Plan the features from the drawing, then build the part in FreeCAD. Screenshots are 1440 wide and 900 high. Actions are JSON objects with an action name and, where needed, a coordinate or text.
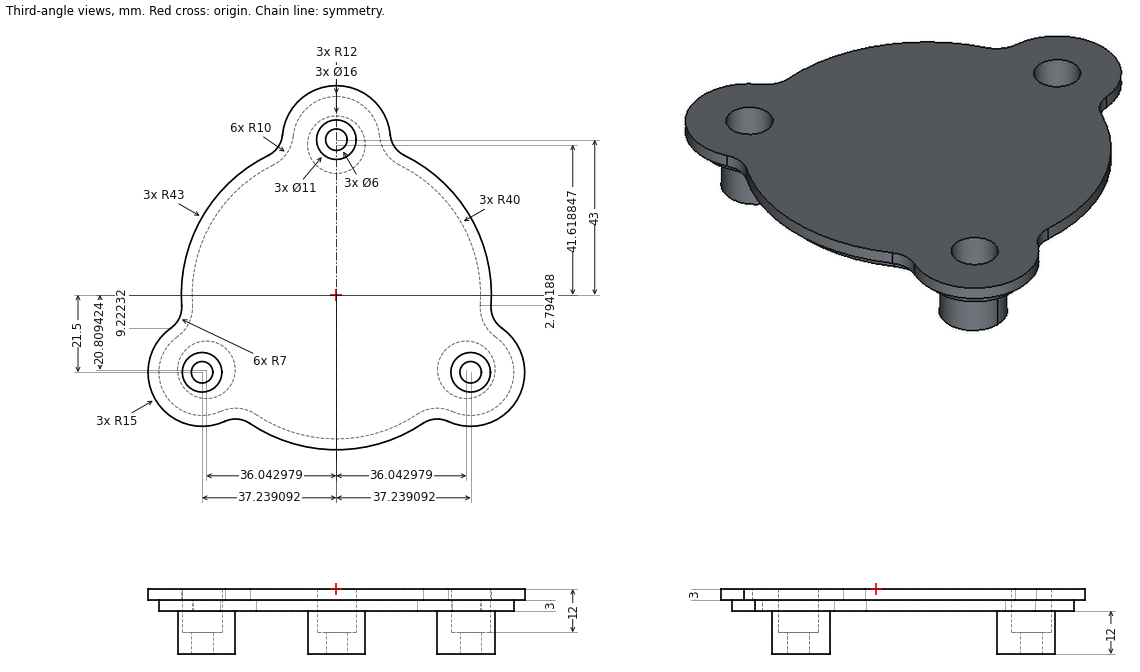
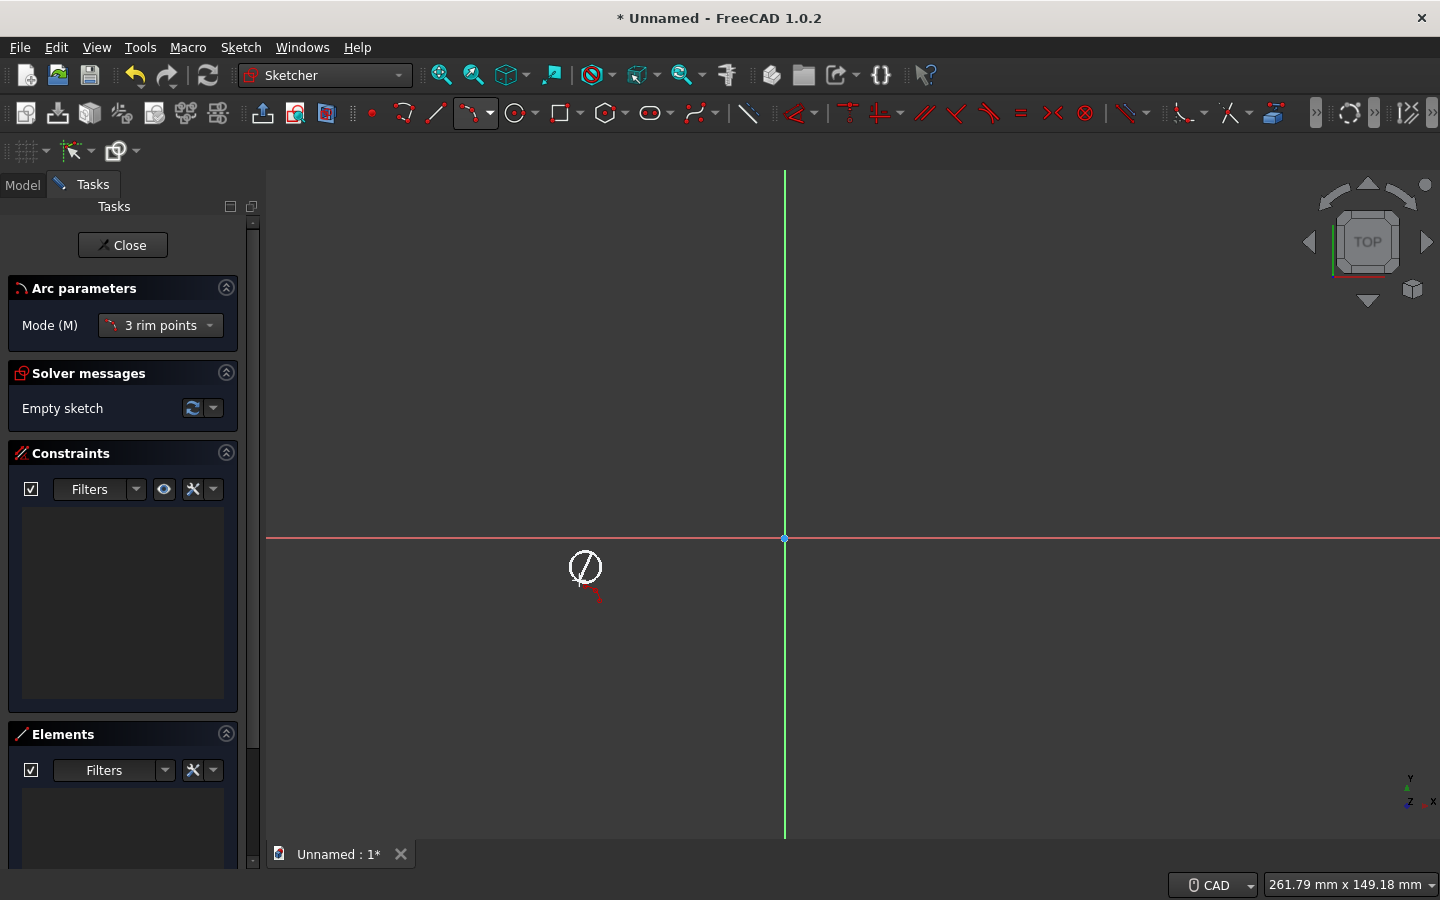
{"action": "scroll", "coordinate": [589, 568], "scroll_direction": "up", "scroll_amount": 7}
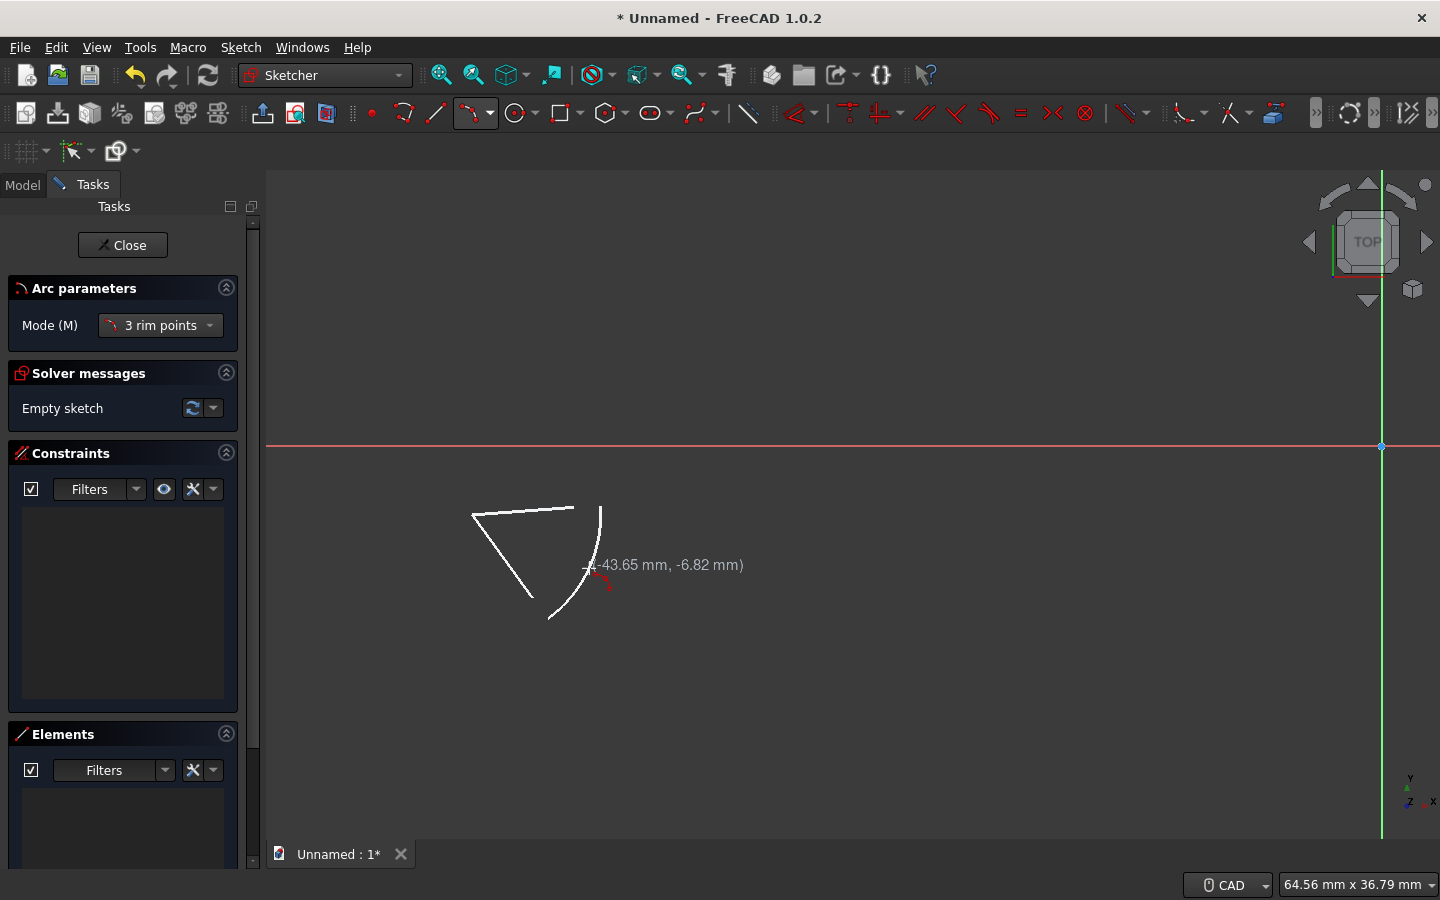
{"action": "left_click", "coordinate": [590, 564]}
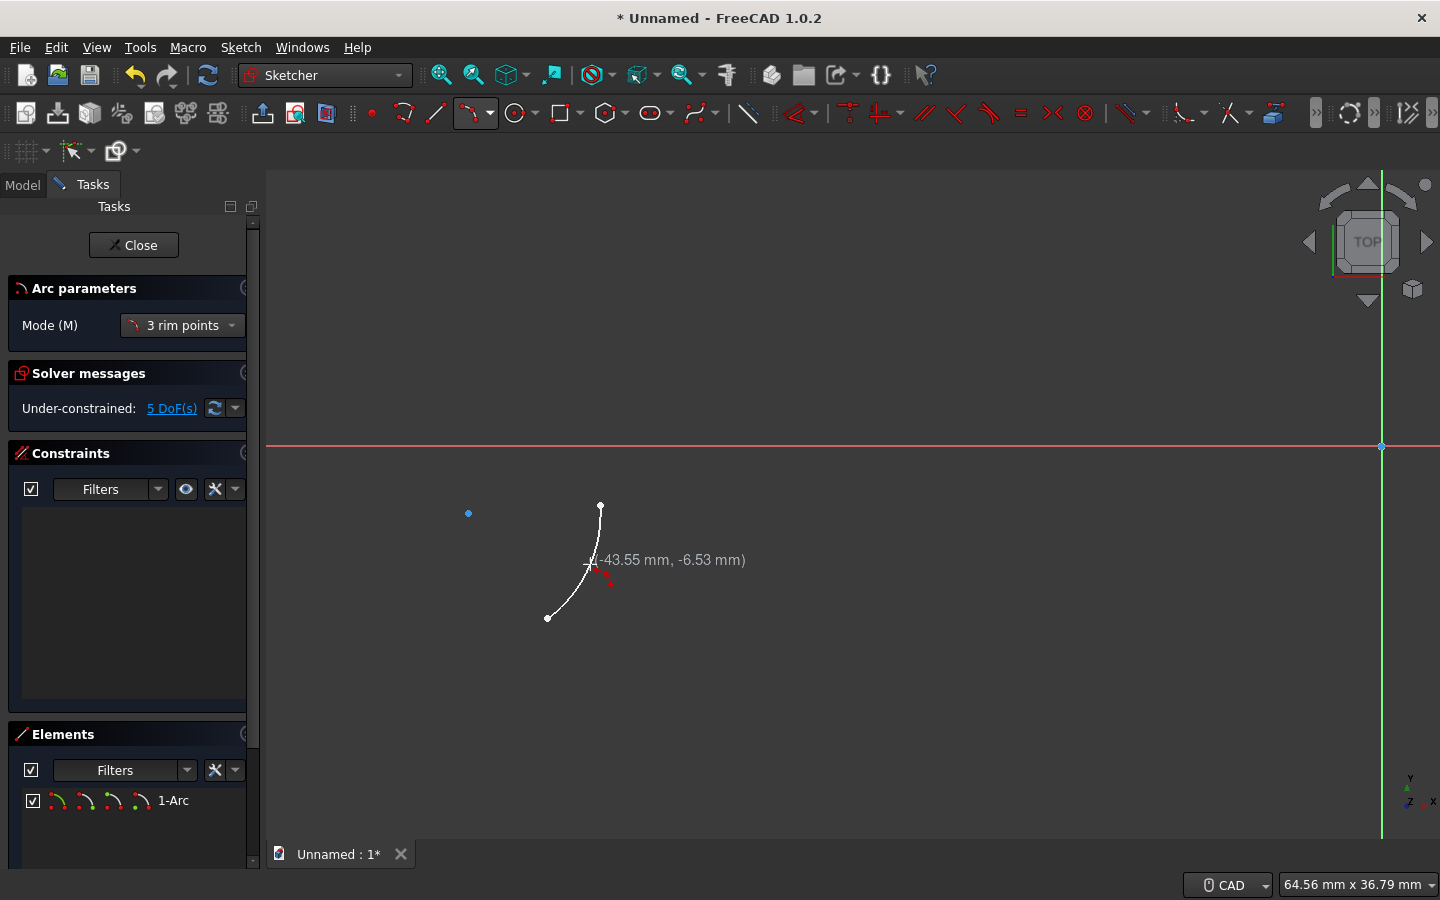
{"action": "scroll", "coordinate": [589, 568], "scroll_direction": "down", "scroll_amount": 7}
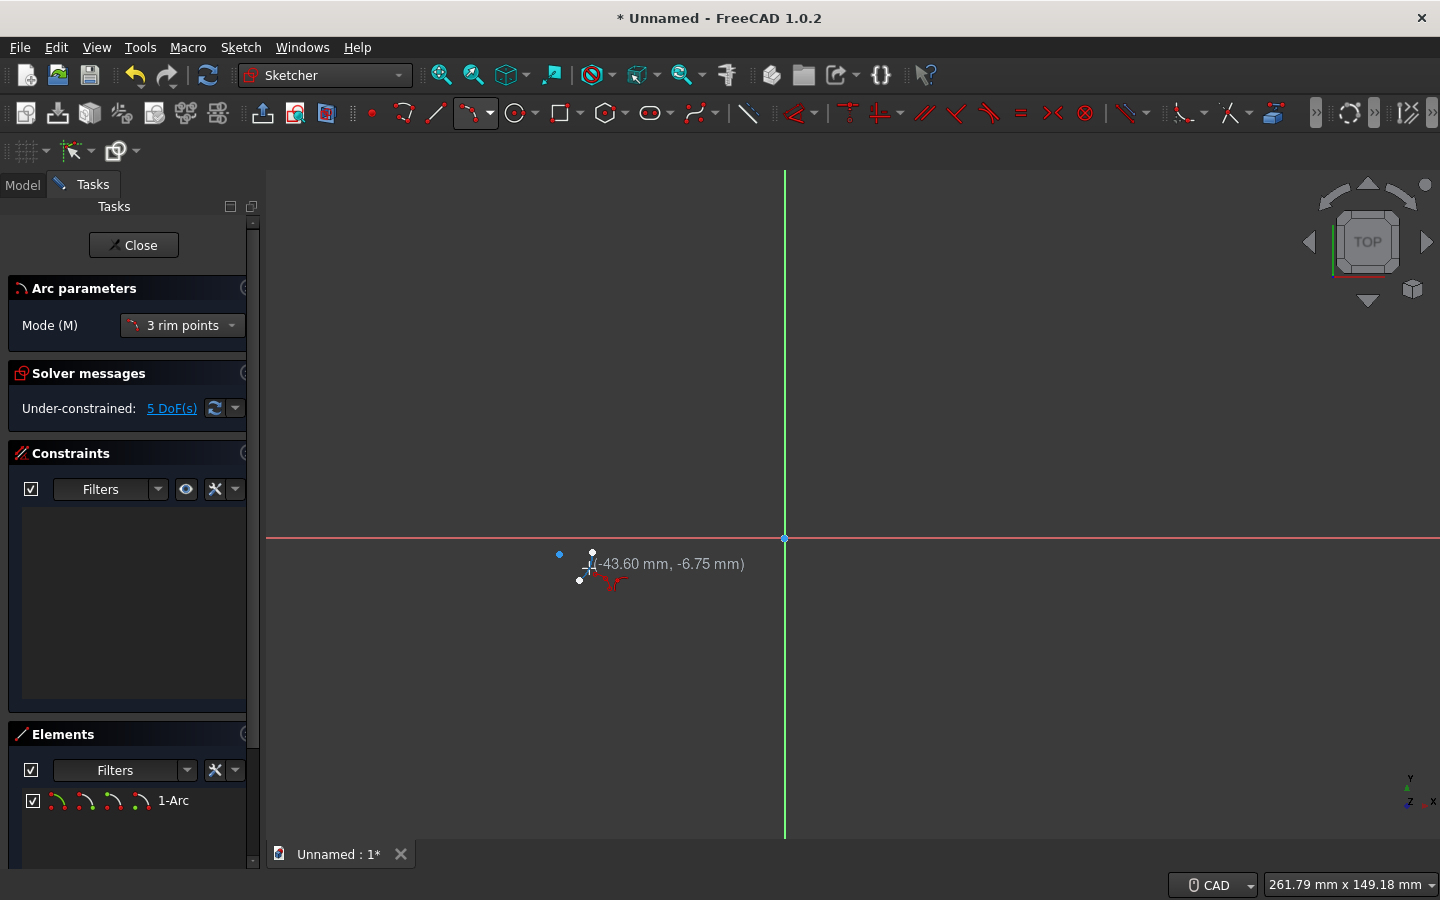
{"action": "left_click", "coordinate": [579, 581]}
{"action": "left_click", "coordinate": [646, 696]}
{"action": "left_click", "coordinate": [559, 668]}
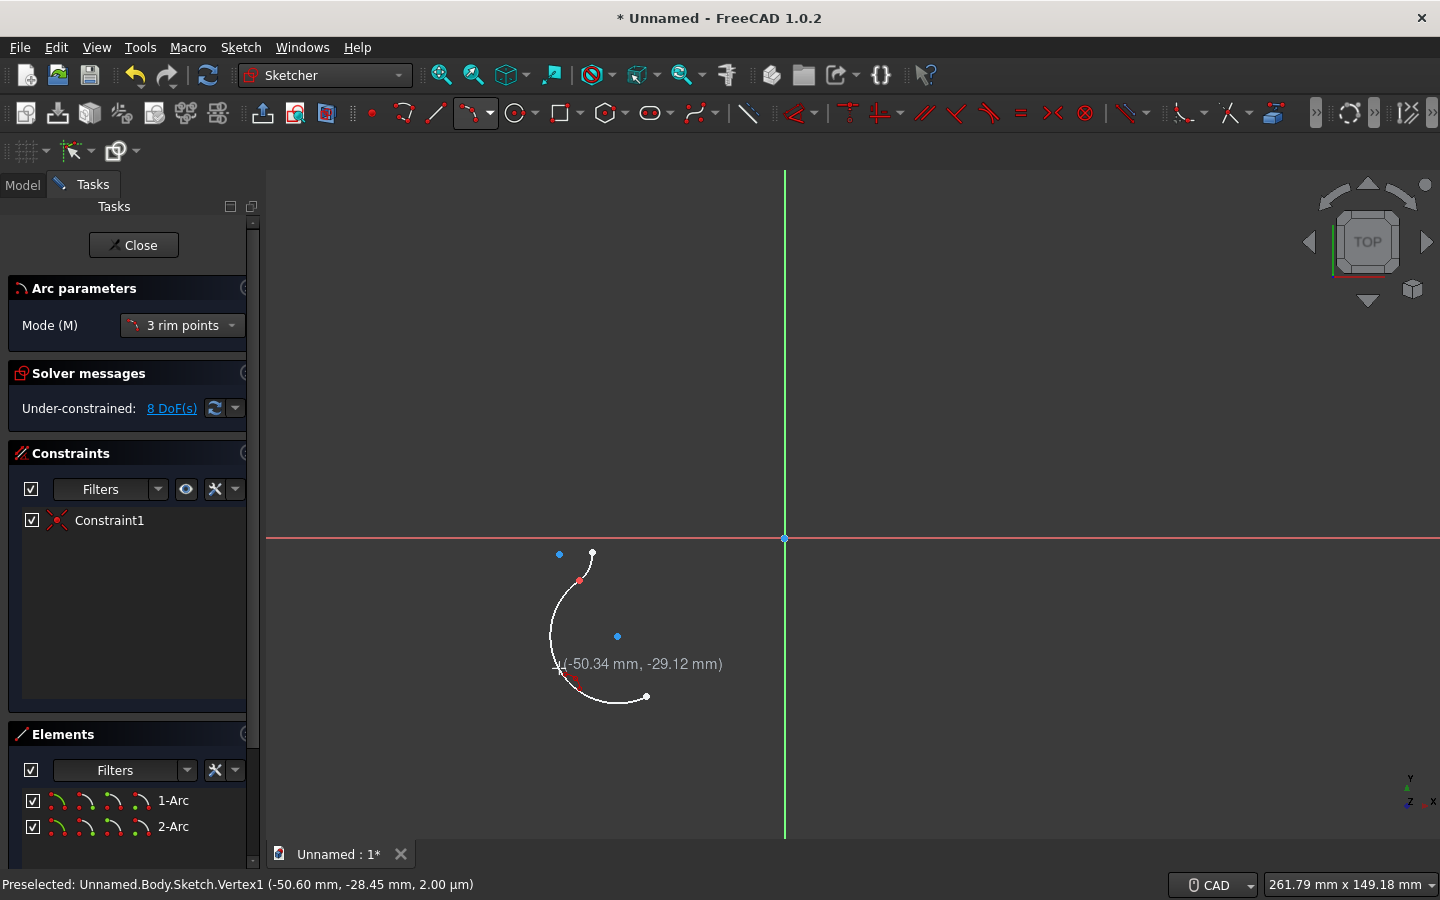
{"action": "left_click", "coordinate": [646, 697]}
{"action": "left_click", "coordinate": [677, 698]}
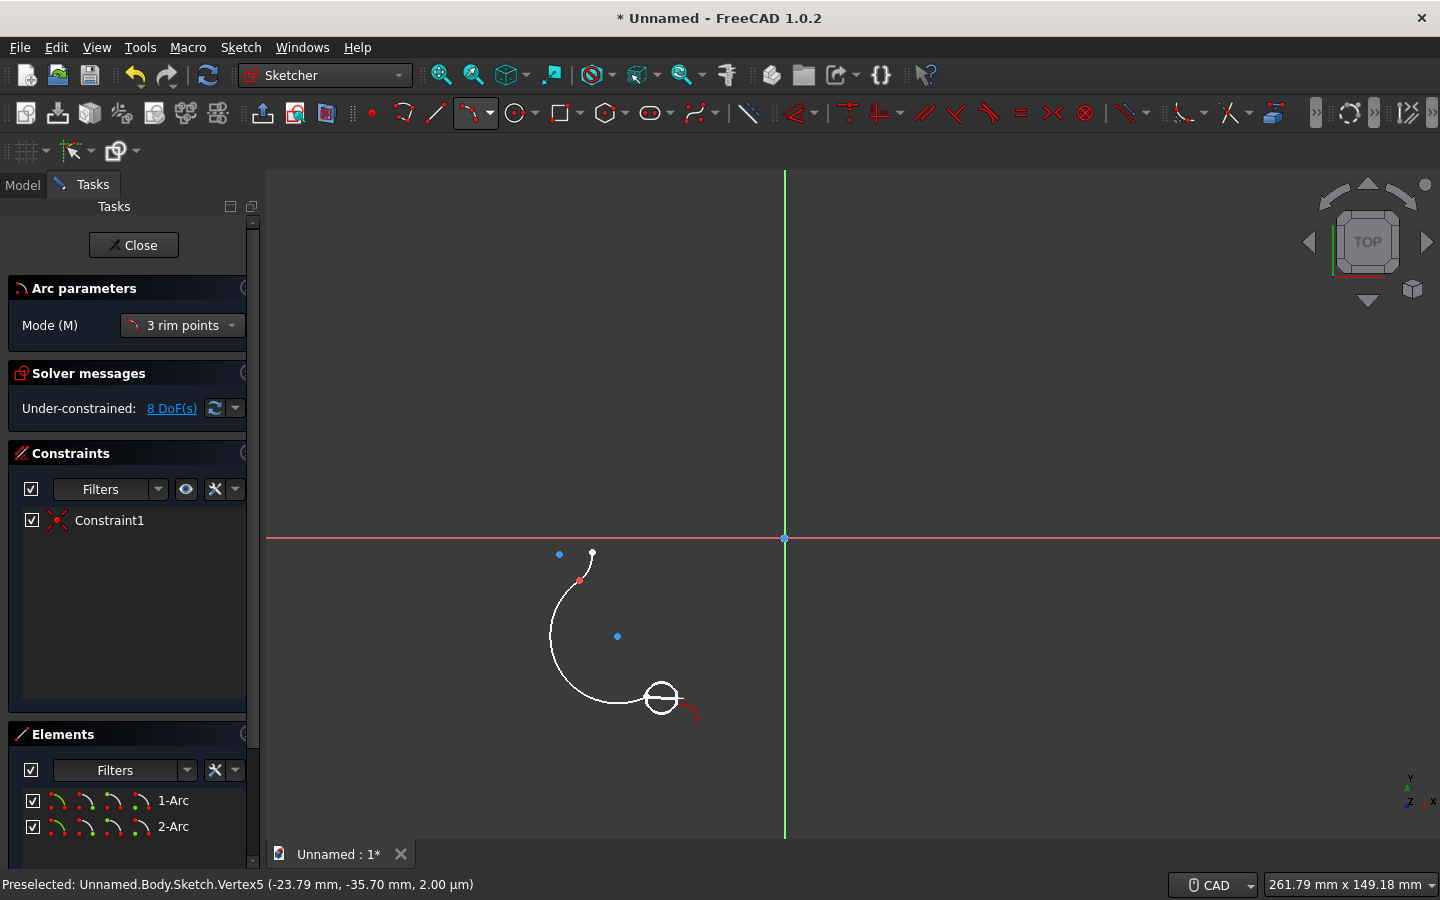
{"action": "scroll", "coordinate": [662, 693], "scroll_direction": "up", "scroll_amount": 7}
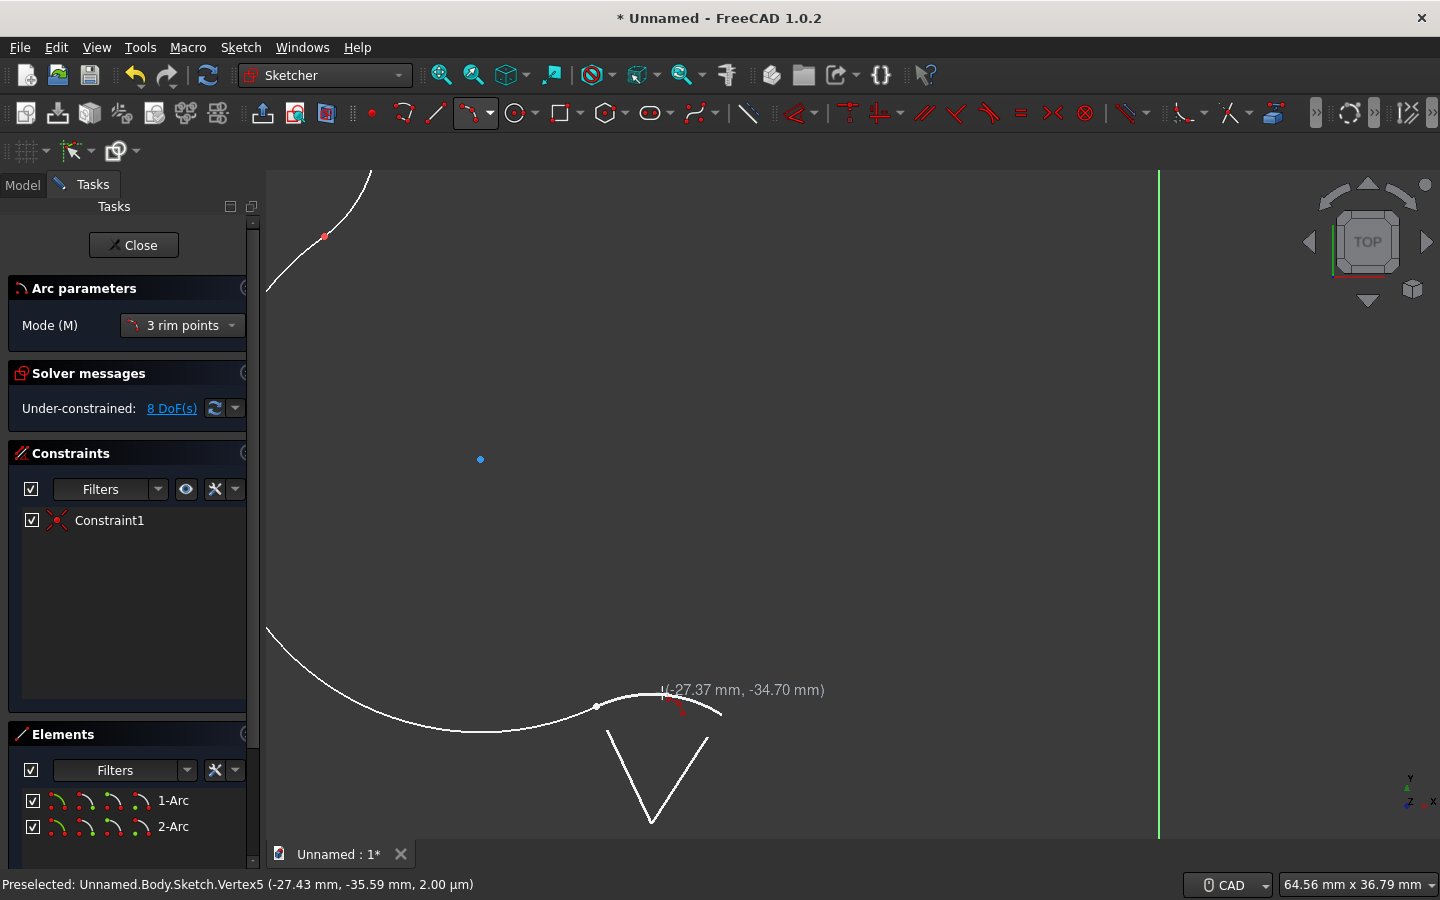
{"action": "left_click", "coordinate": [660, 691]}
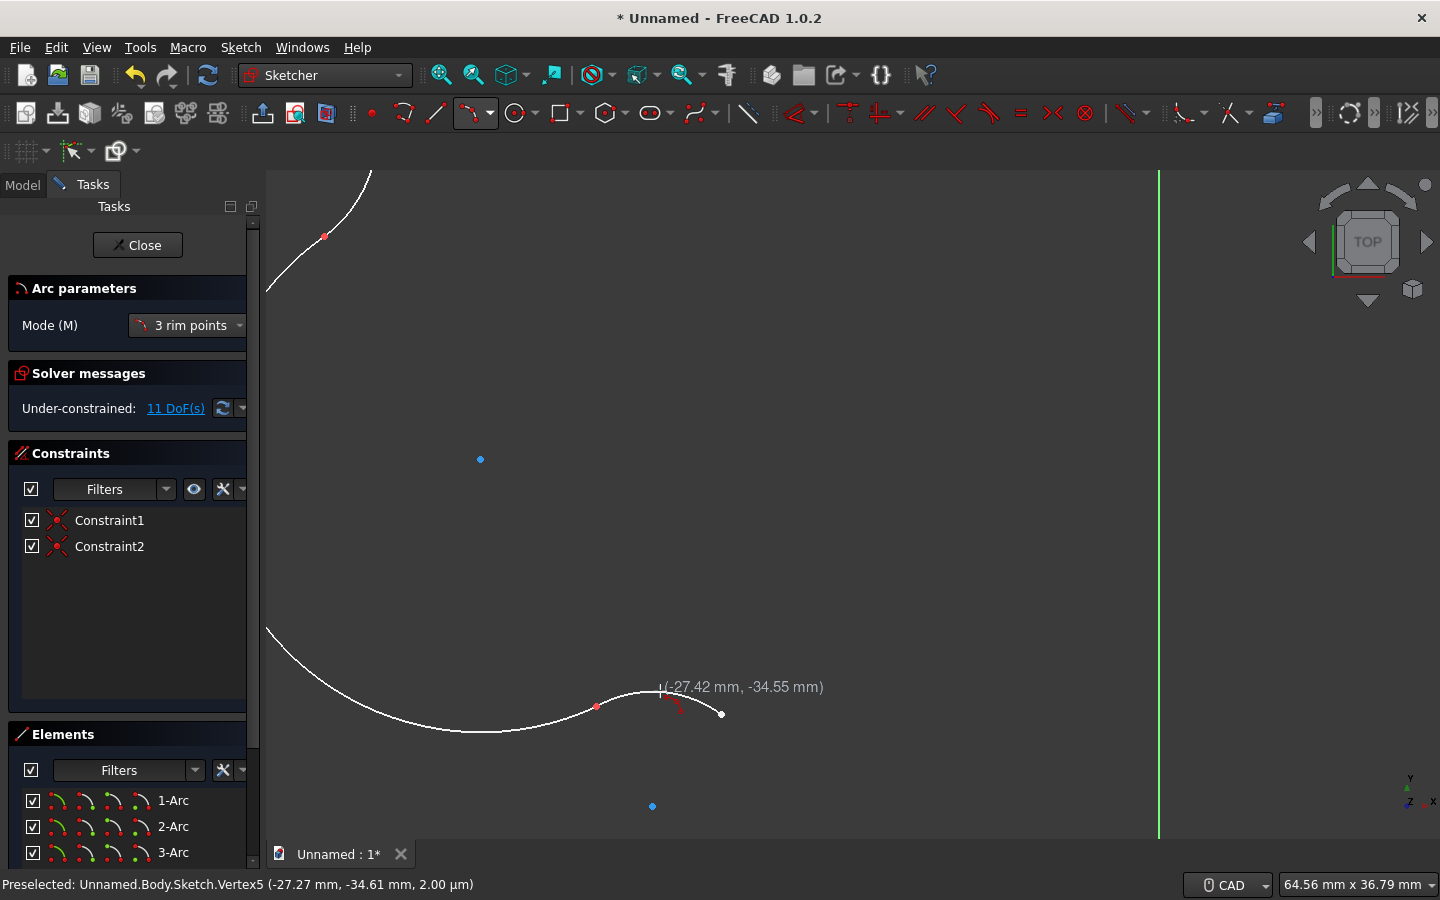
{"action": "scroll", "coordinate": [662, 693], "scroll_direction": "down", "scroll_amount": 7}